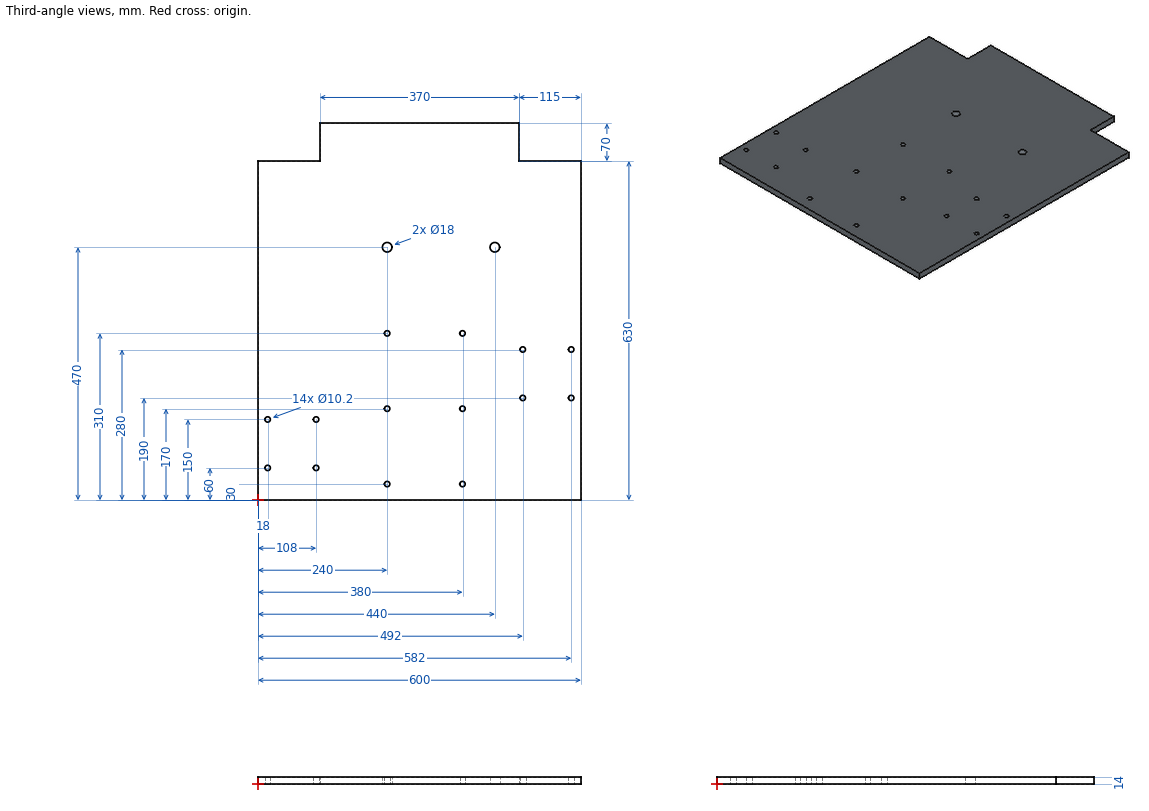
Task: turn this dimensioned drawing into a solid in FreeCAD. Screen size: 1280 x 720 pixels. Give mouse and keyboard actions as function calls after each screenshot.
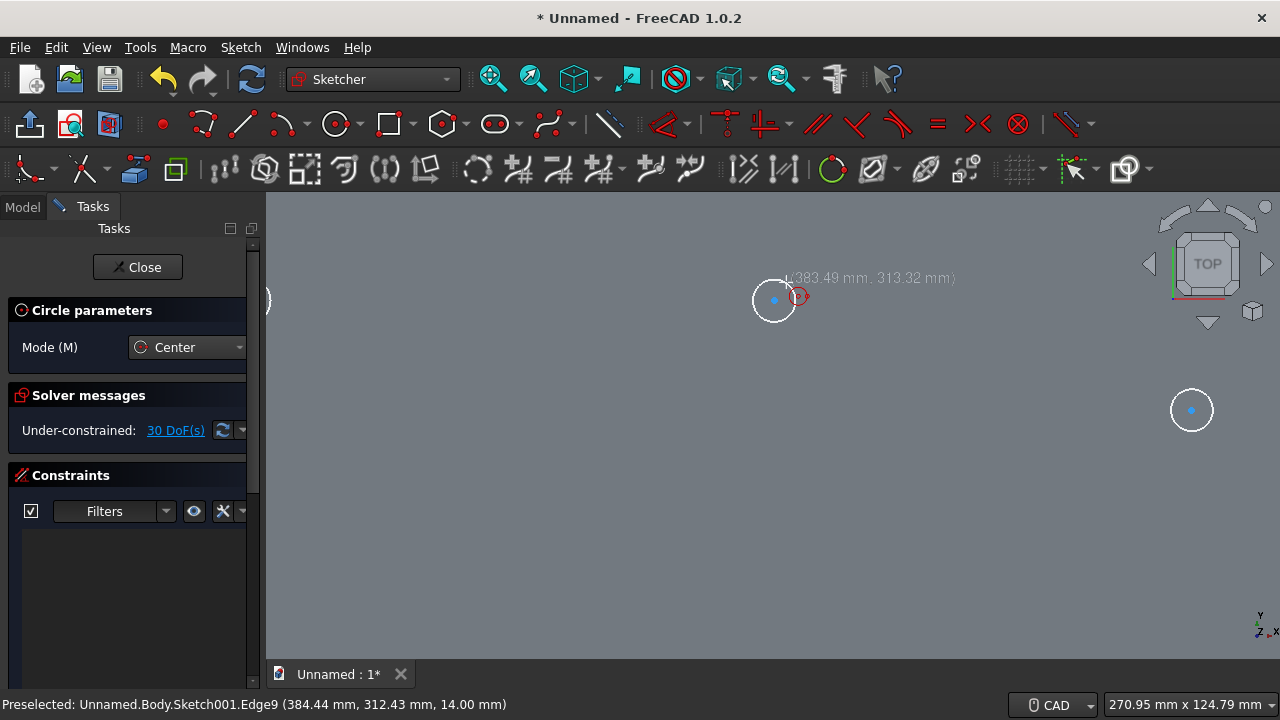
scroll(788, 281, down, 7)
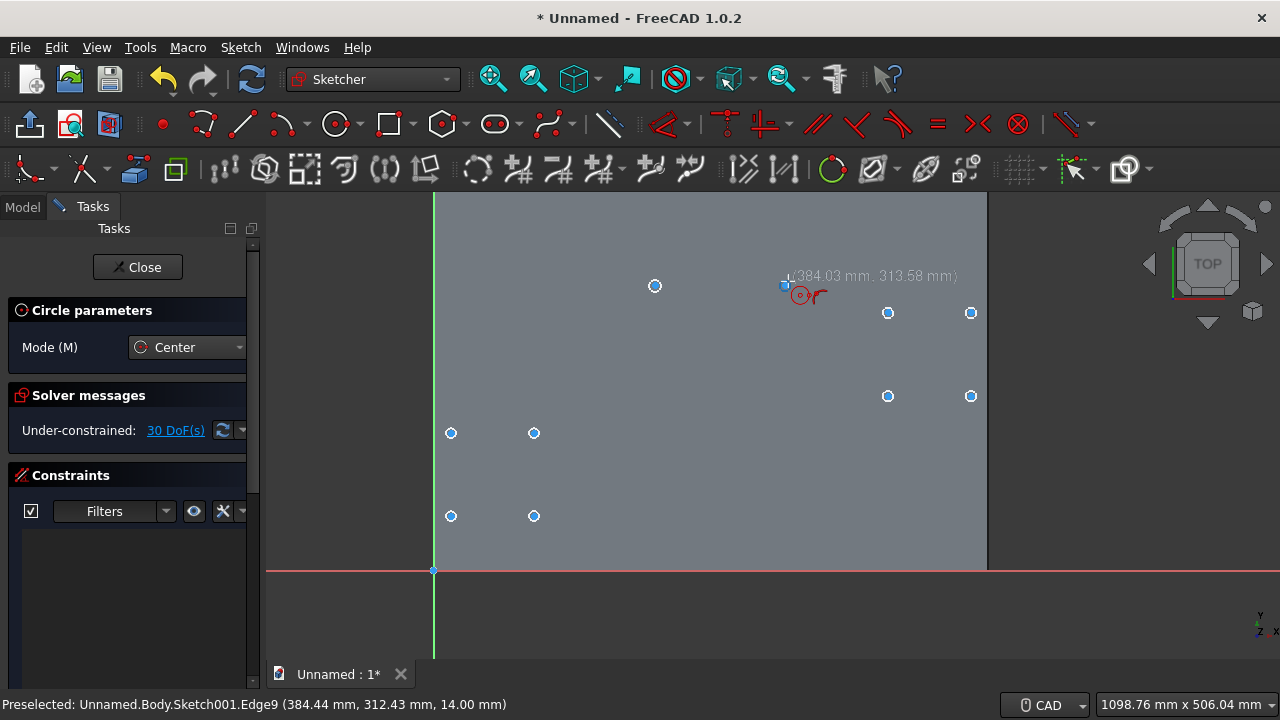
scroll(655, 414, up, 8)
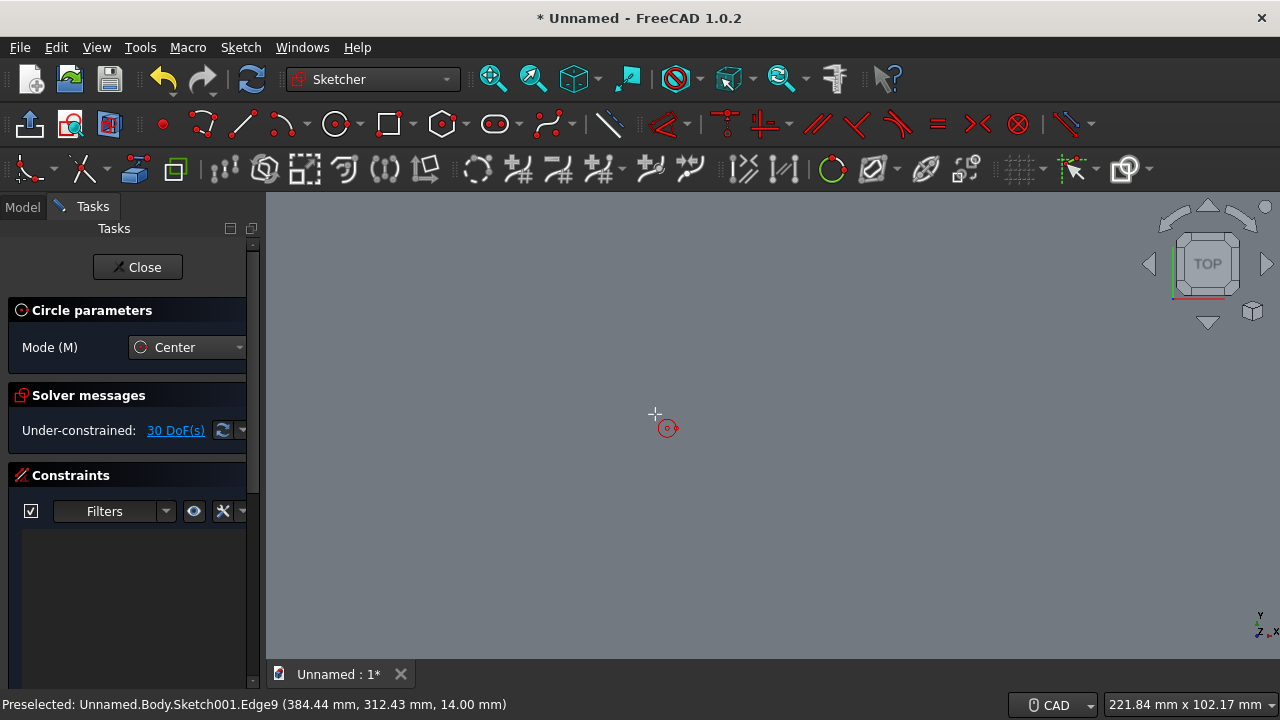
scroll(655, 415, down, 8)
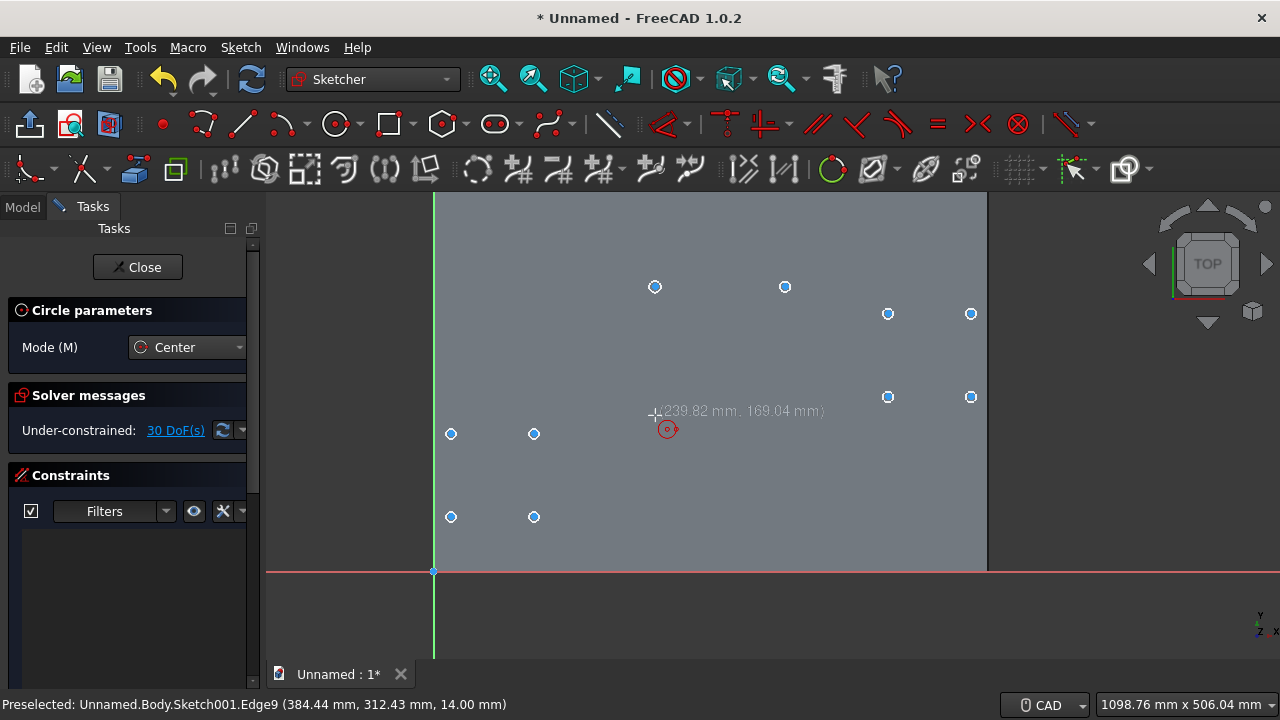
click(655, 415)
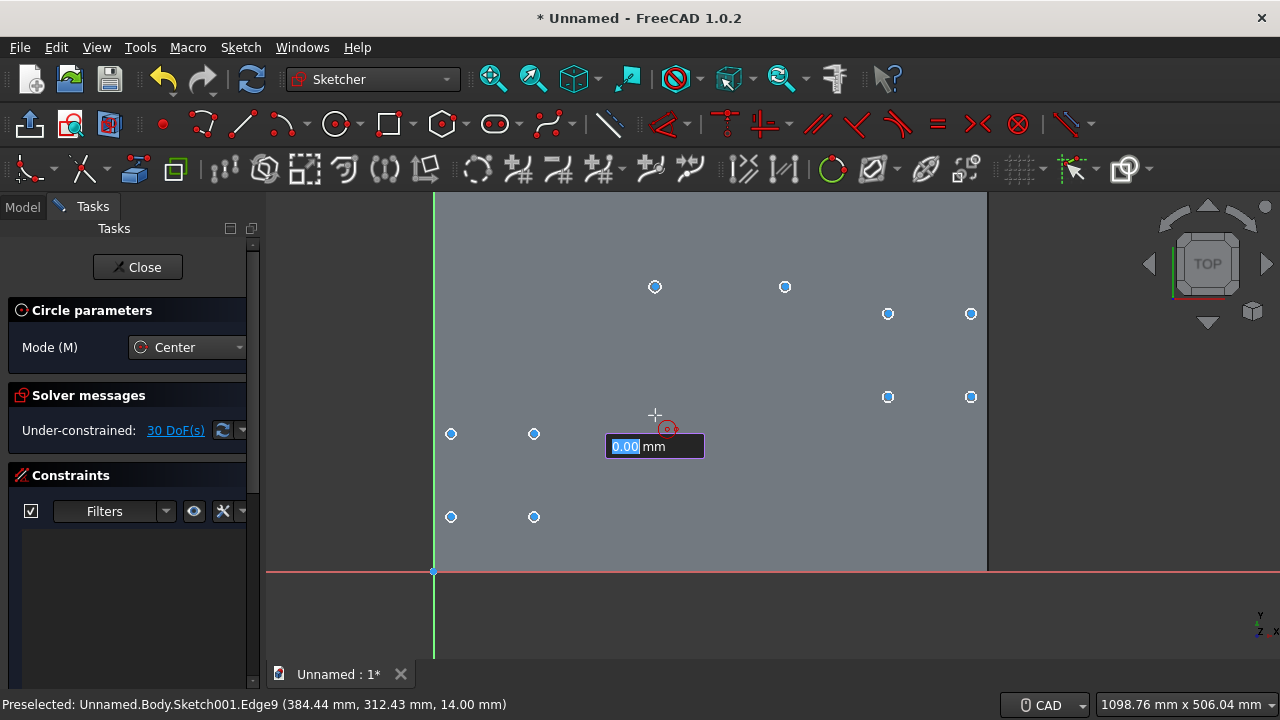
scroll(659, 411, up, 7)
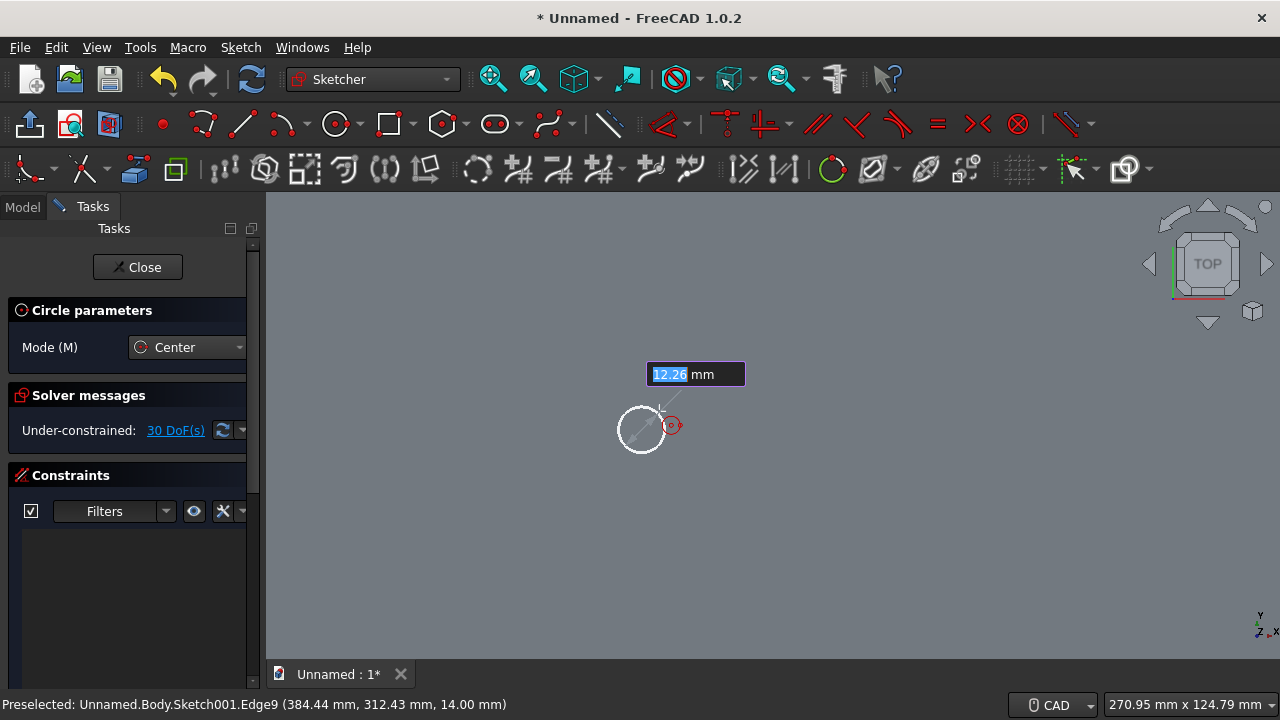
click(657, 411)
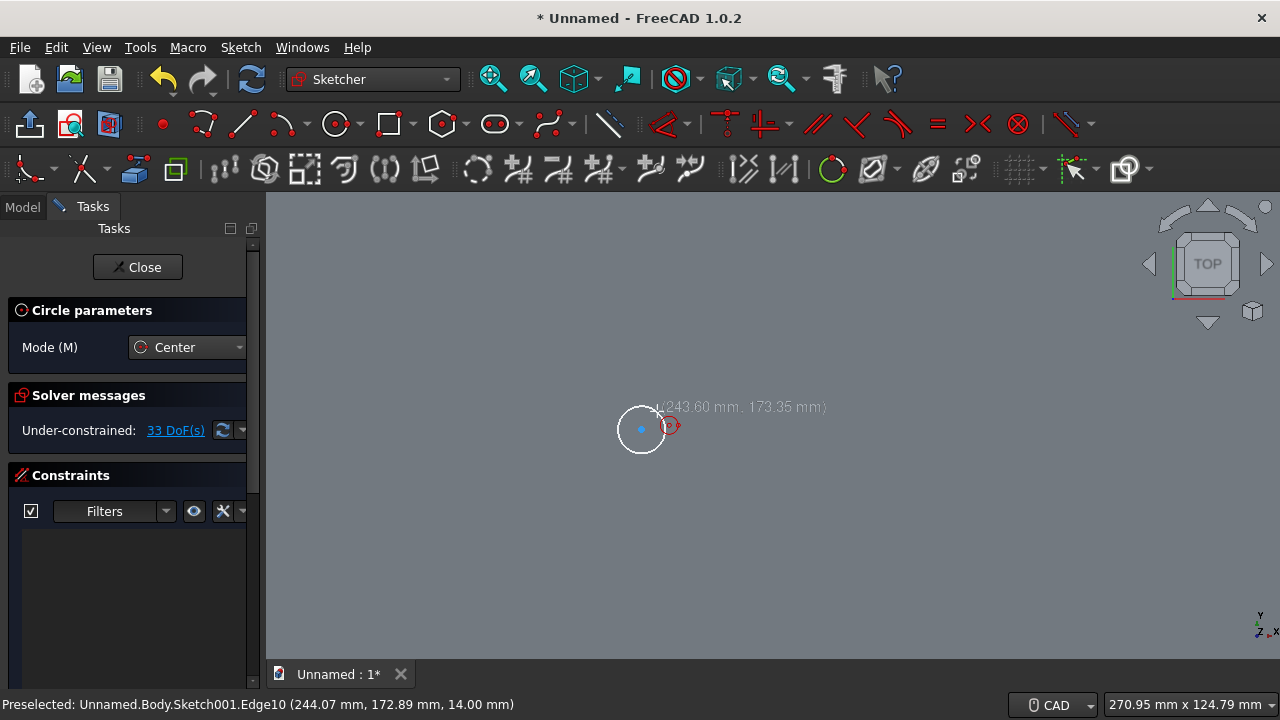
scroll(659, 411, down, 7)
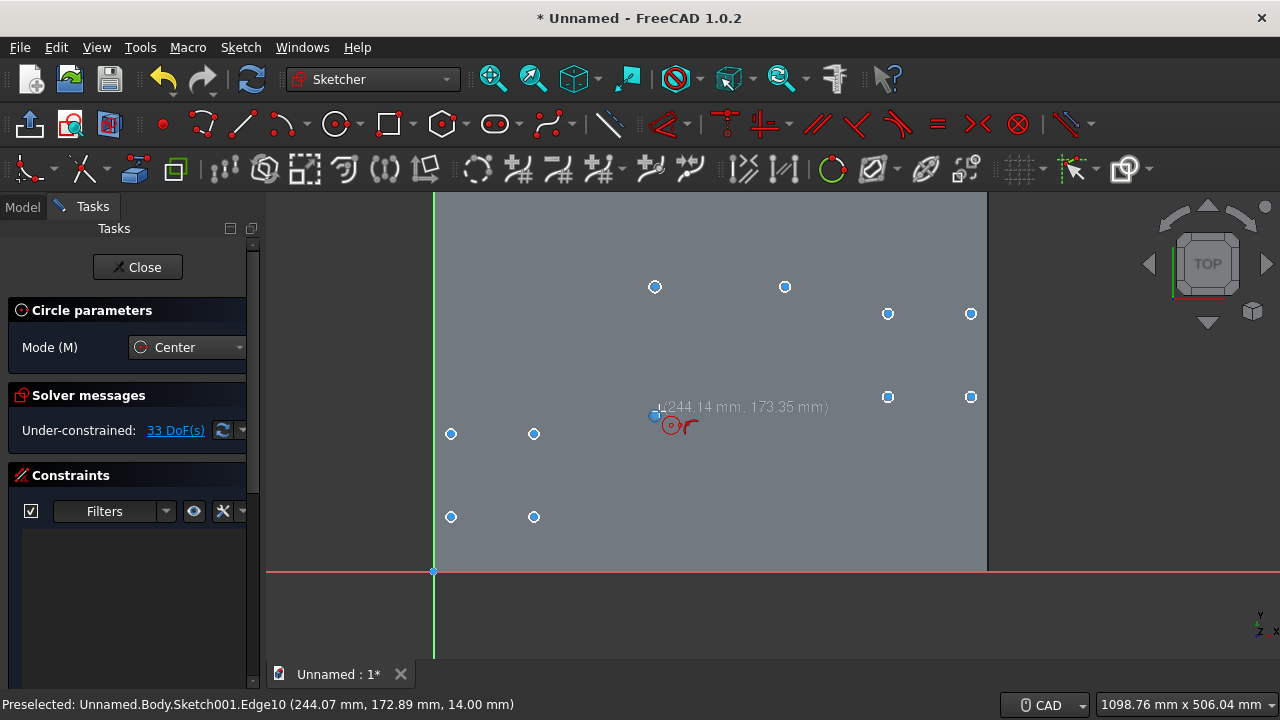
scroll(785, 415, up, 8)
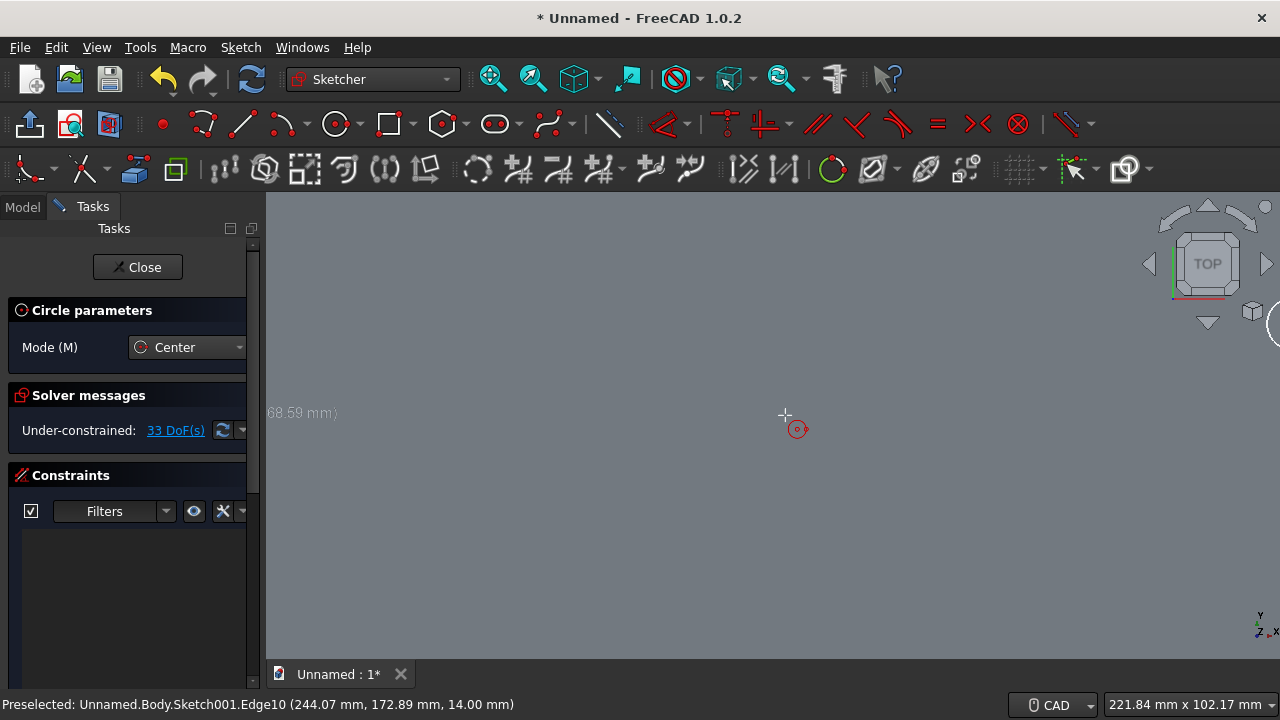
scroll(785, 415, down, 8)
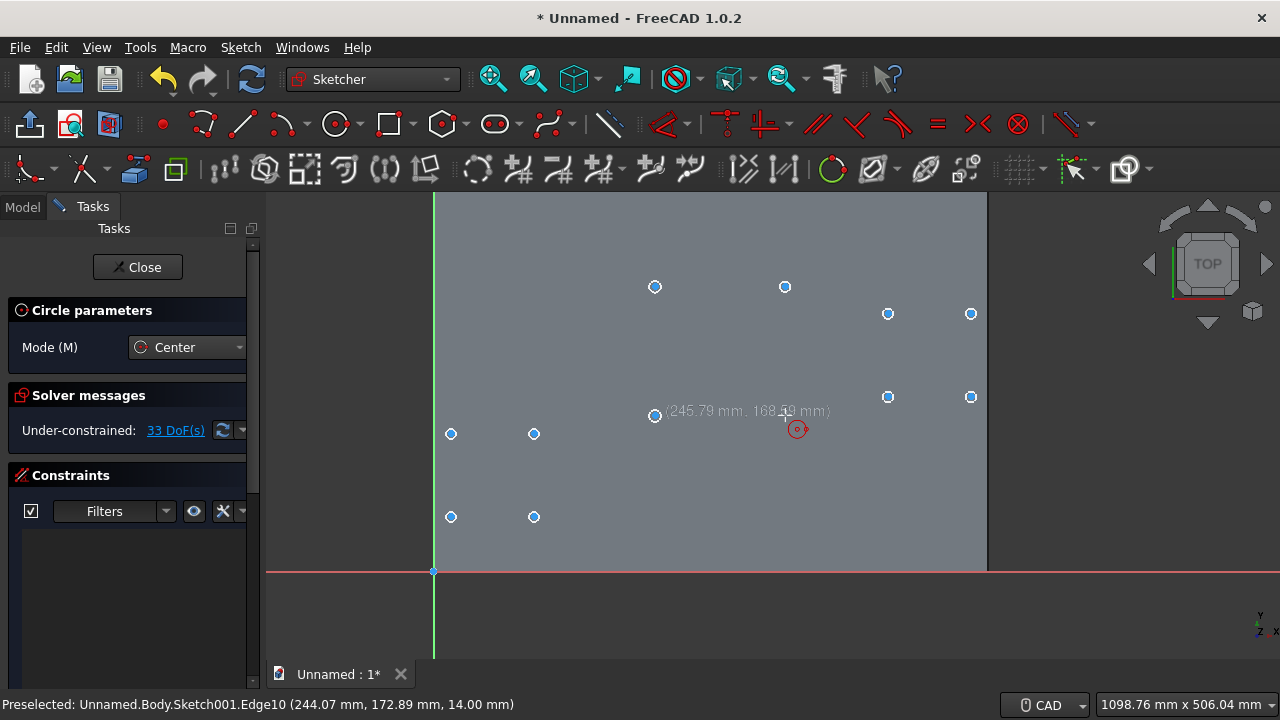
click(785, 415)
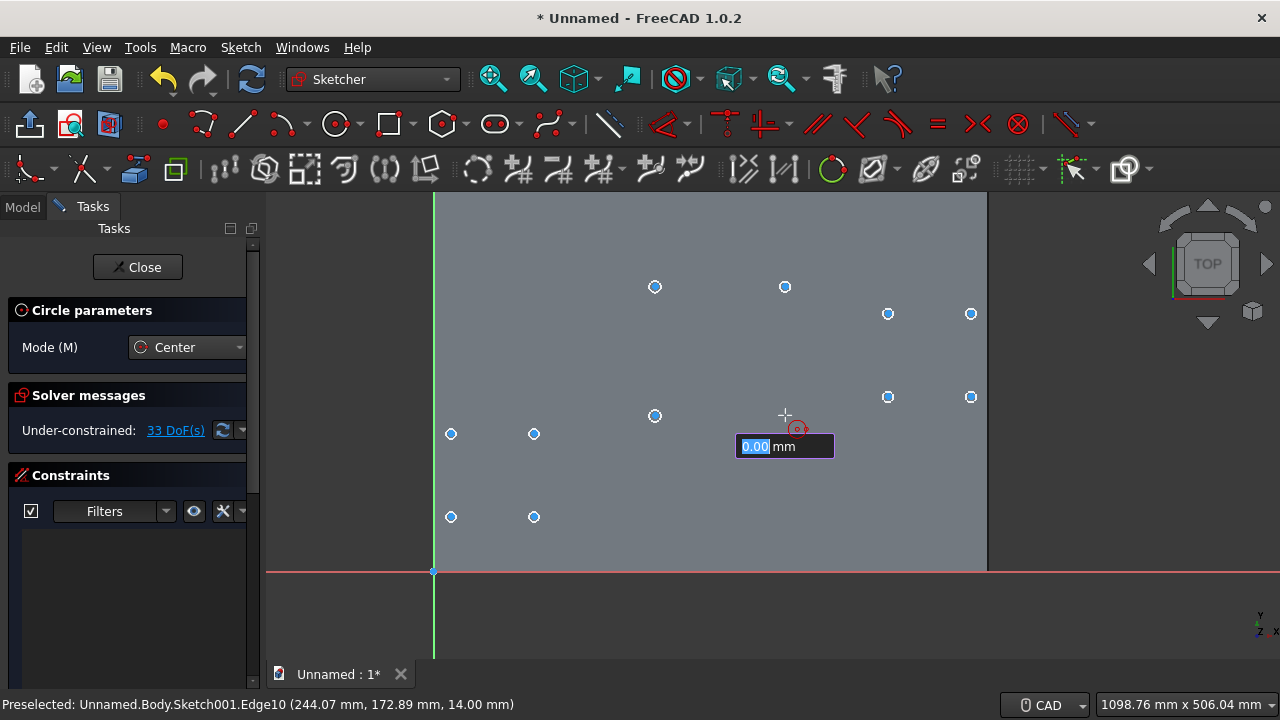
scroll(788, 411, up, 7)